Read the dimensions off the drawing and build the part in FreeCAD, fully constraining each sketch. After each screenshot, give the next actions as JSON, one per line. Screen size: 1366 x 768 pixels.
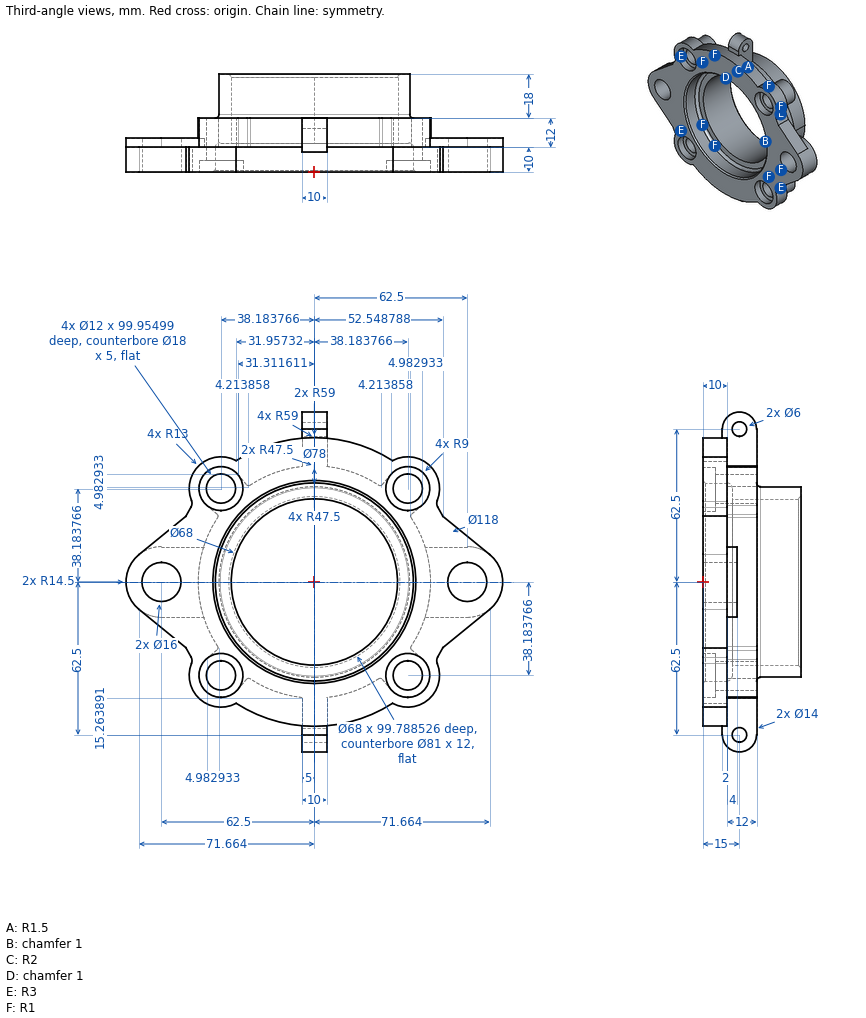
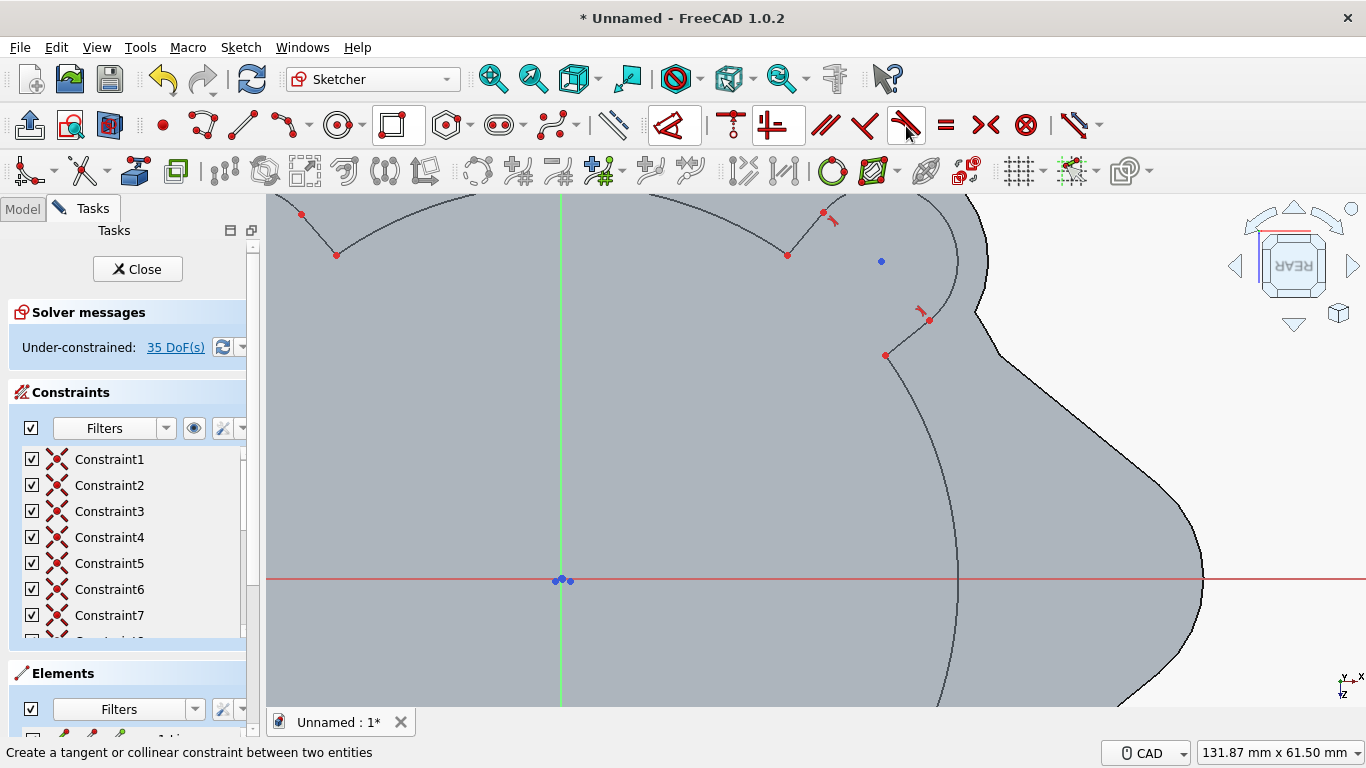
{"action": "left_click", "coordinate": [326, 243]}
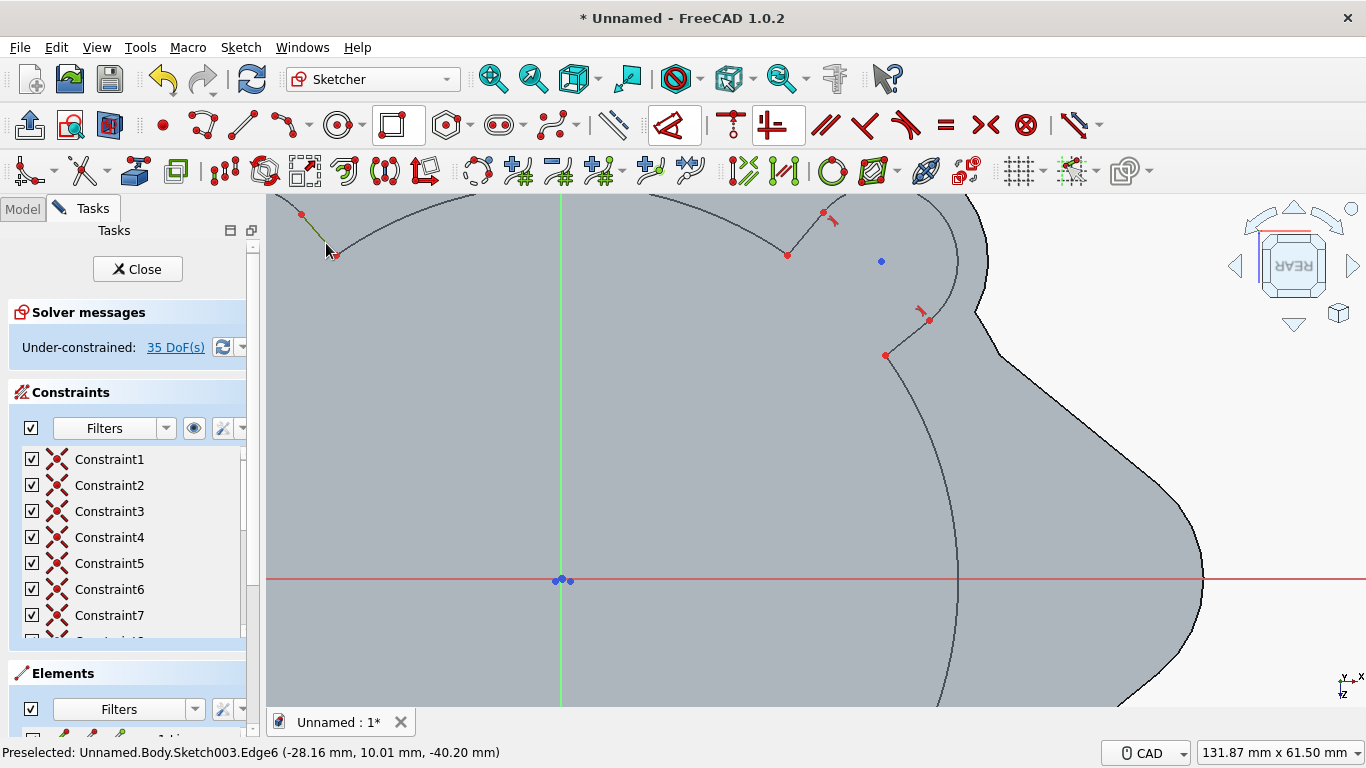
{"action": "scroll", "coordinate": [899, 346], "scroll_direction": "down", "scroll_amount": 4}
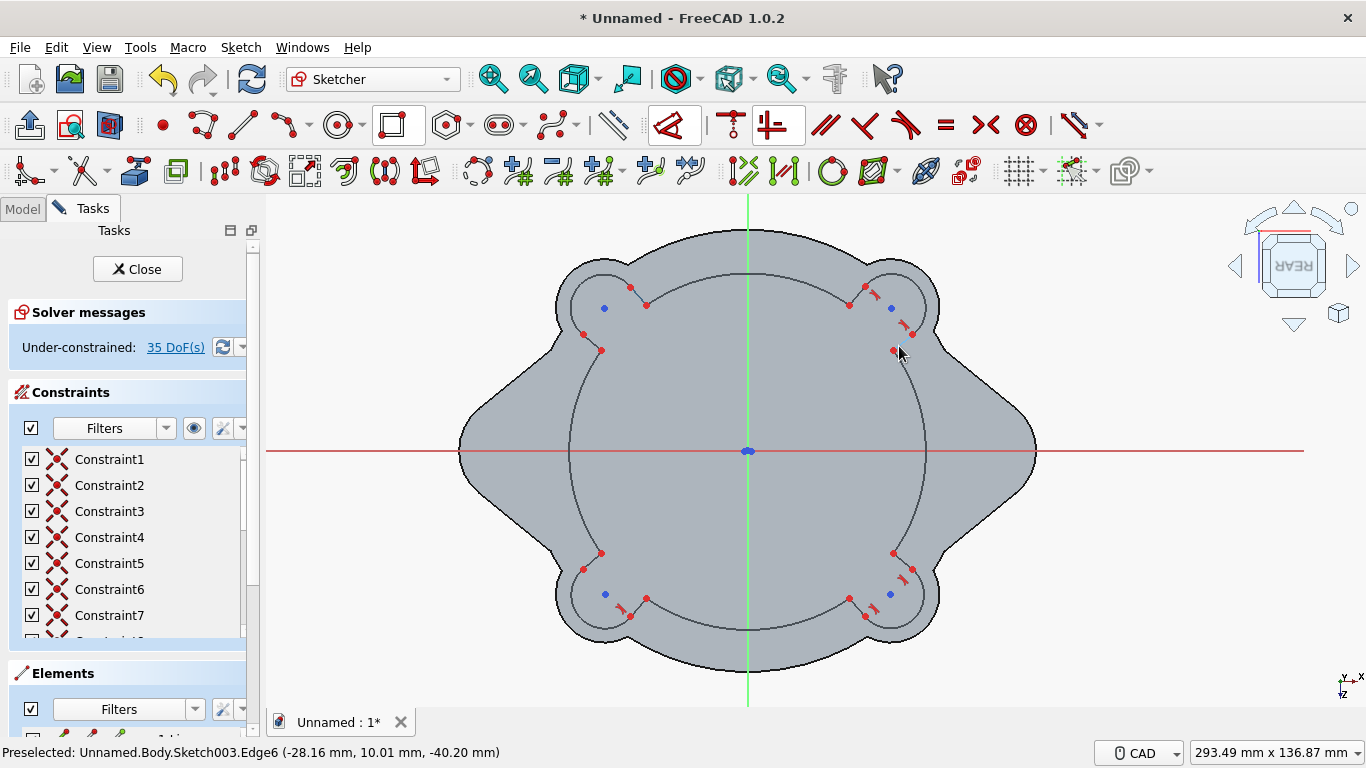
{"action": "left_click", "coordinate": [601, 275]}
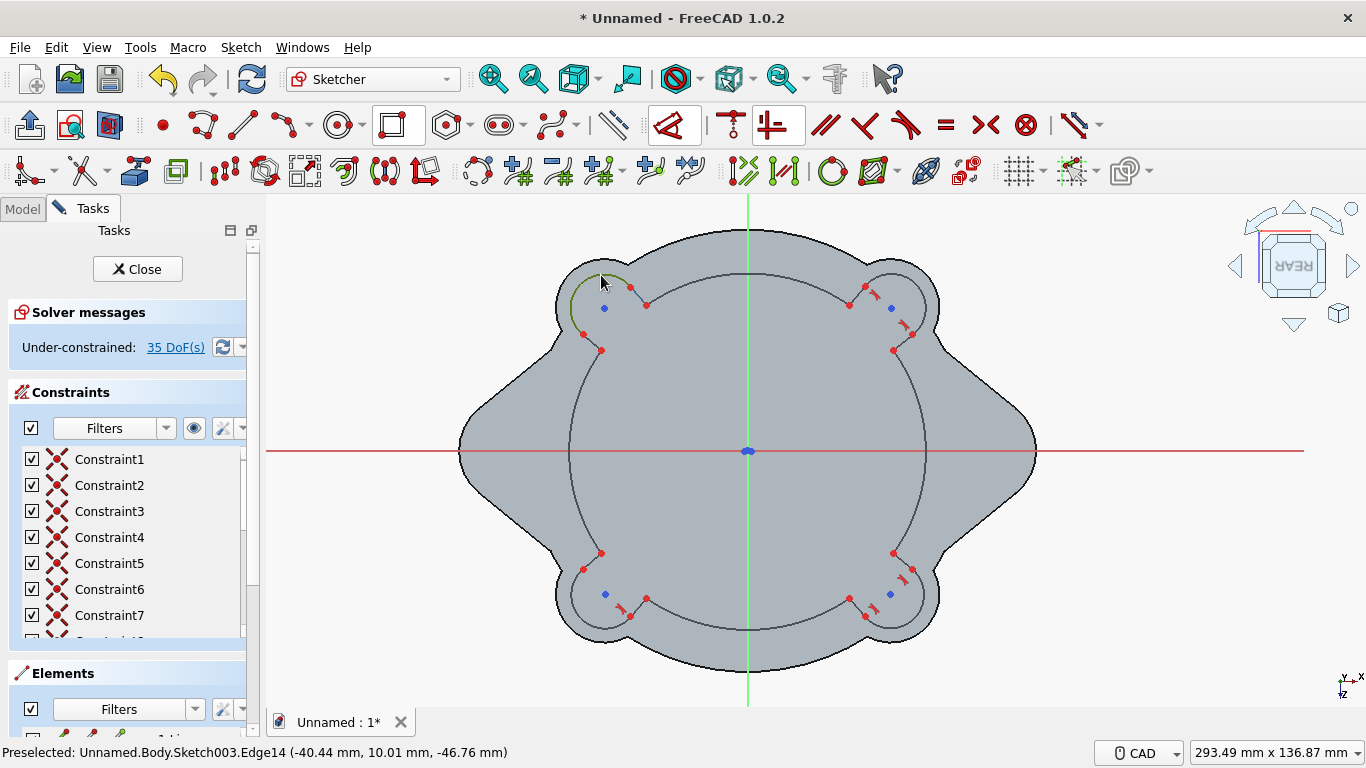
{"action": "left_click", "coordinate": [906, 126]}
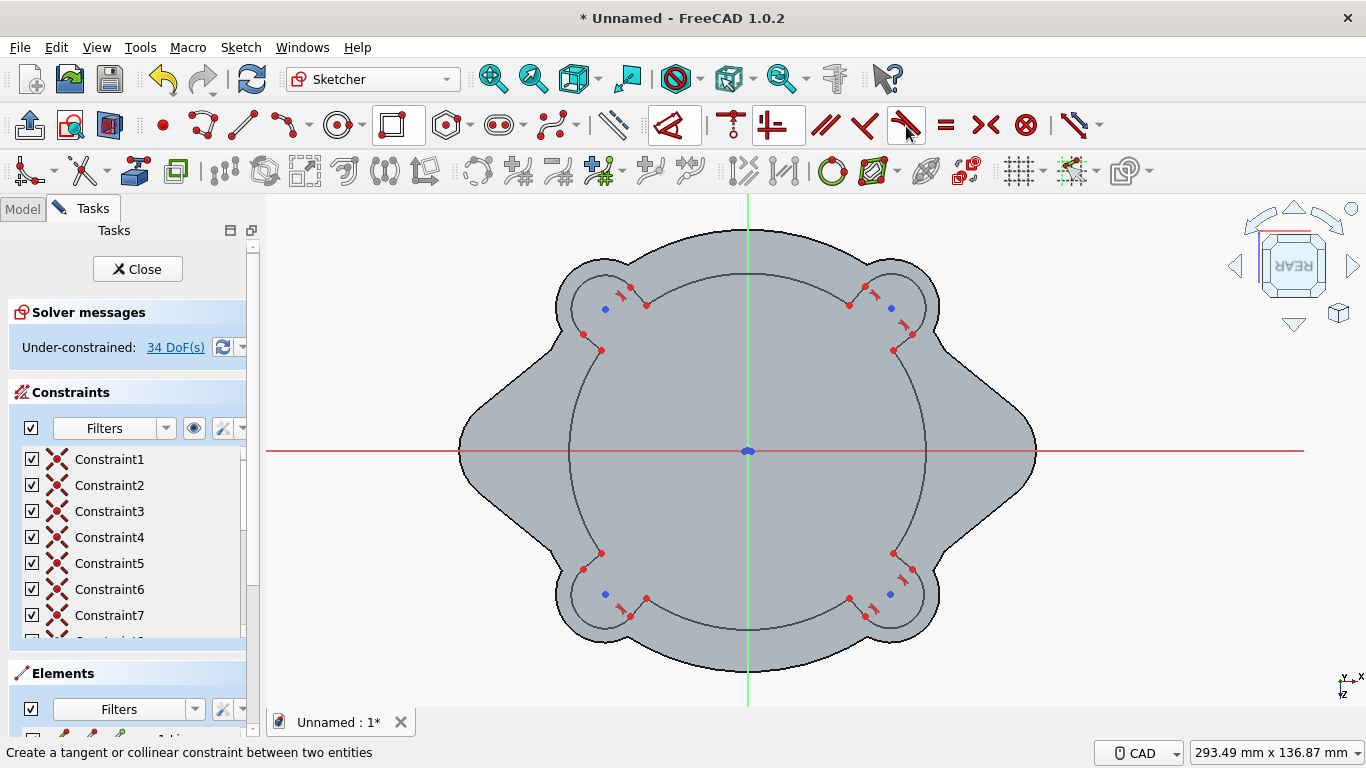
{"action": "scroll", "coordinate": [590, 341], "scroll_direction": "up", "scroll_amount": 2}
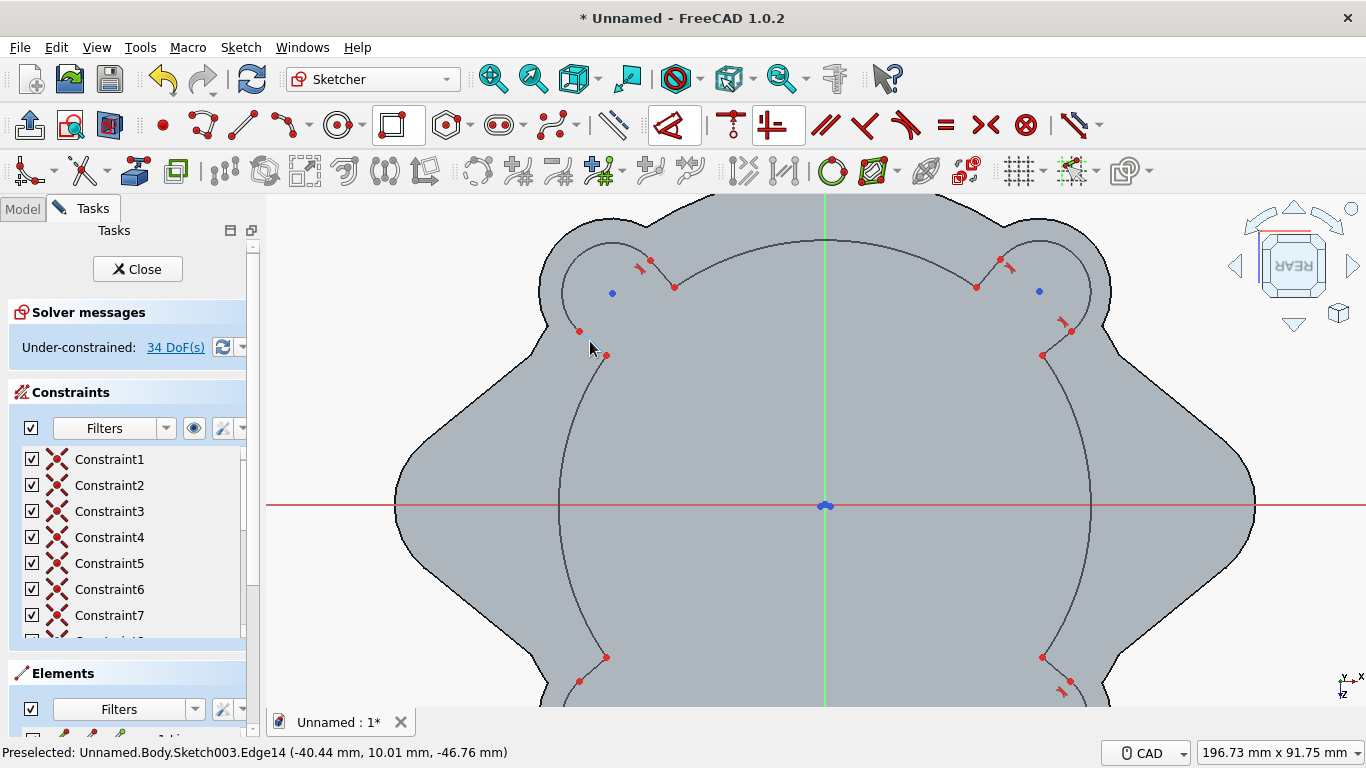
{"action": "left_click", "coordinate": [590, 341]}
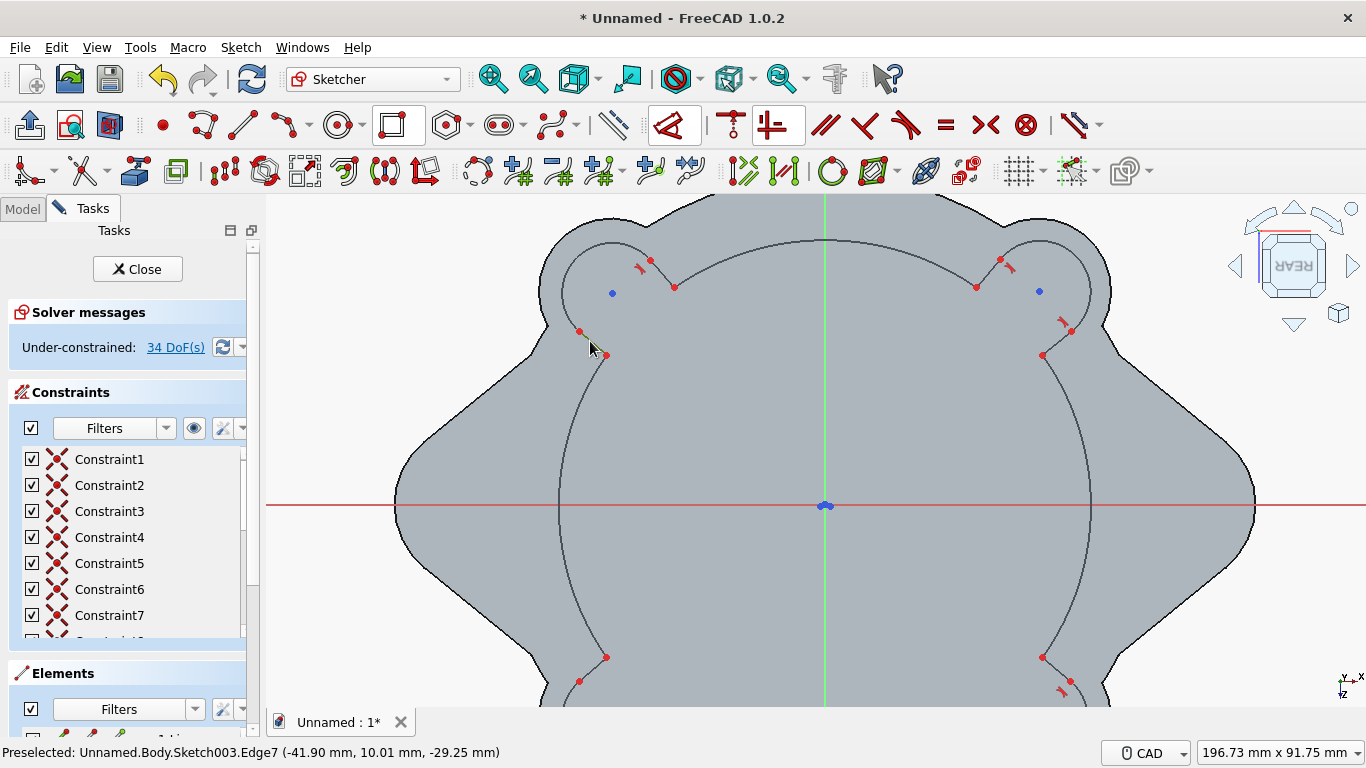
{"action": "left_click", "coordinate": [606, 243]}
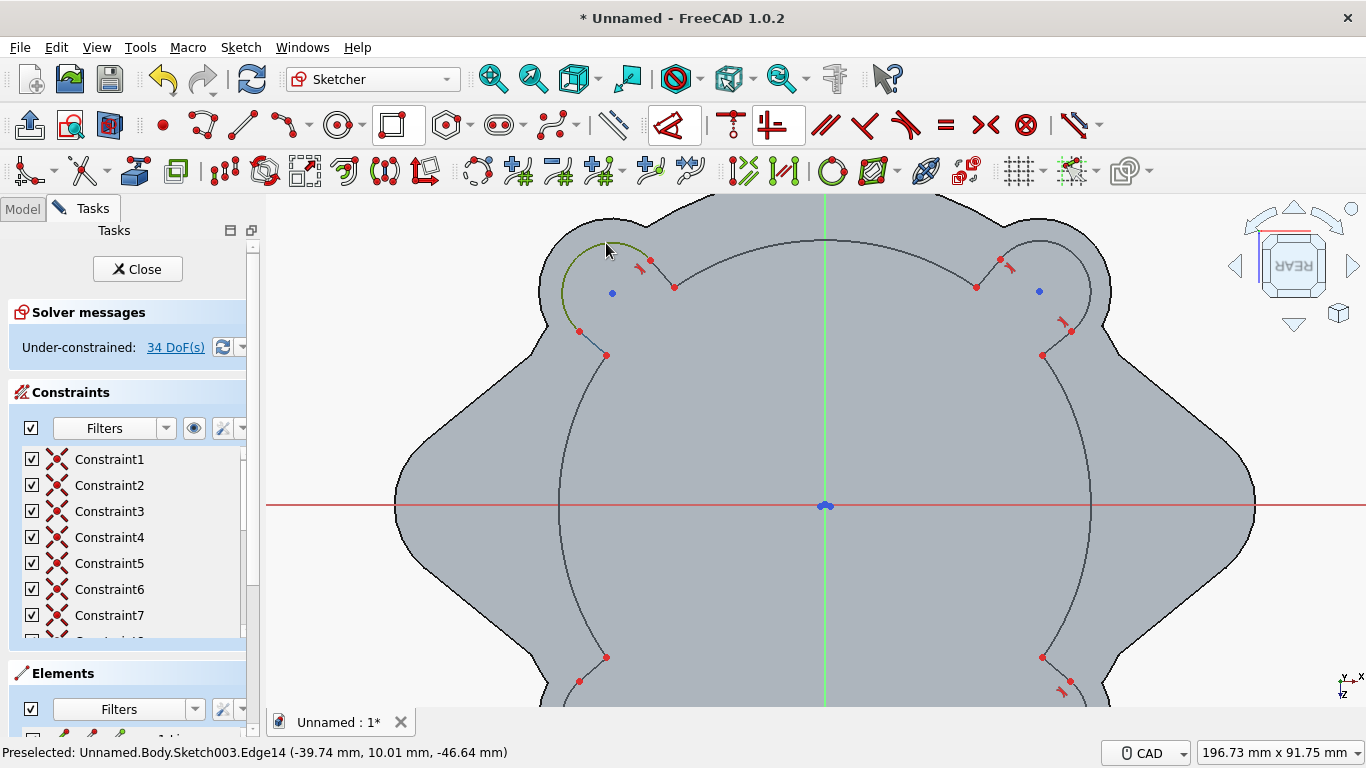
{"action": "left_click", "coordinate": [906, 126]}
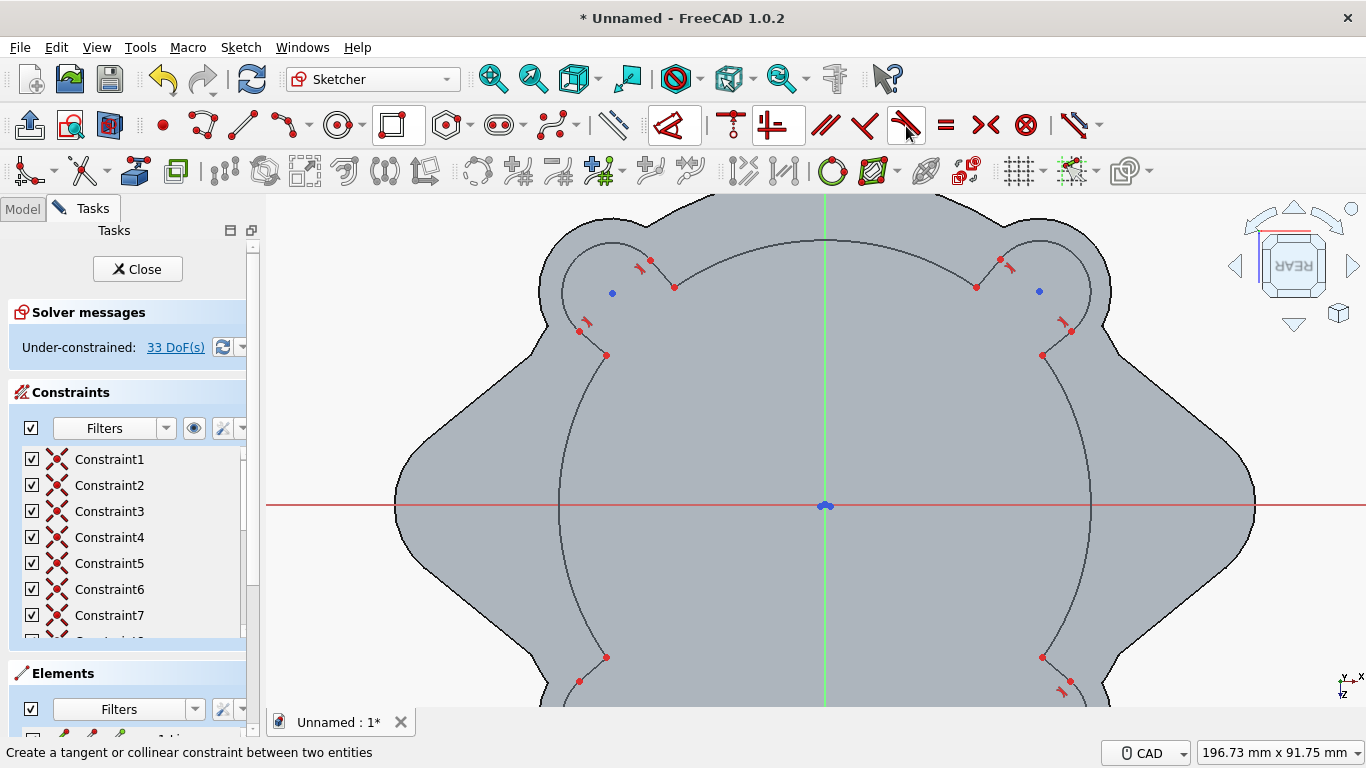
{"action": "scroll", "coordinate": [599, 665], "scroll_direction": "up", "scroll_amount": 2}